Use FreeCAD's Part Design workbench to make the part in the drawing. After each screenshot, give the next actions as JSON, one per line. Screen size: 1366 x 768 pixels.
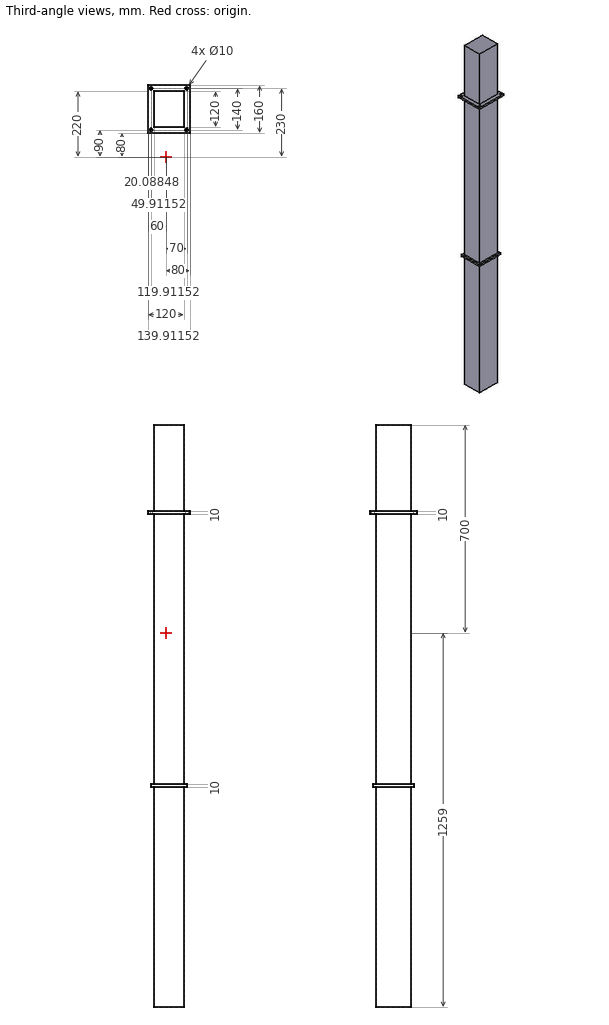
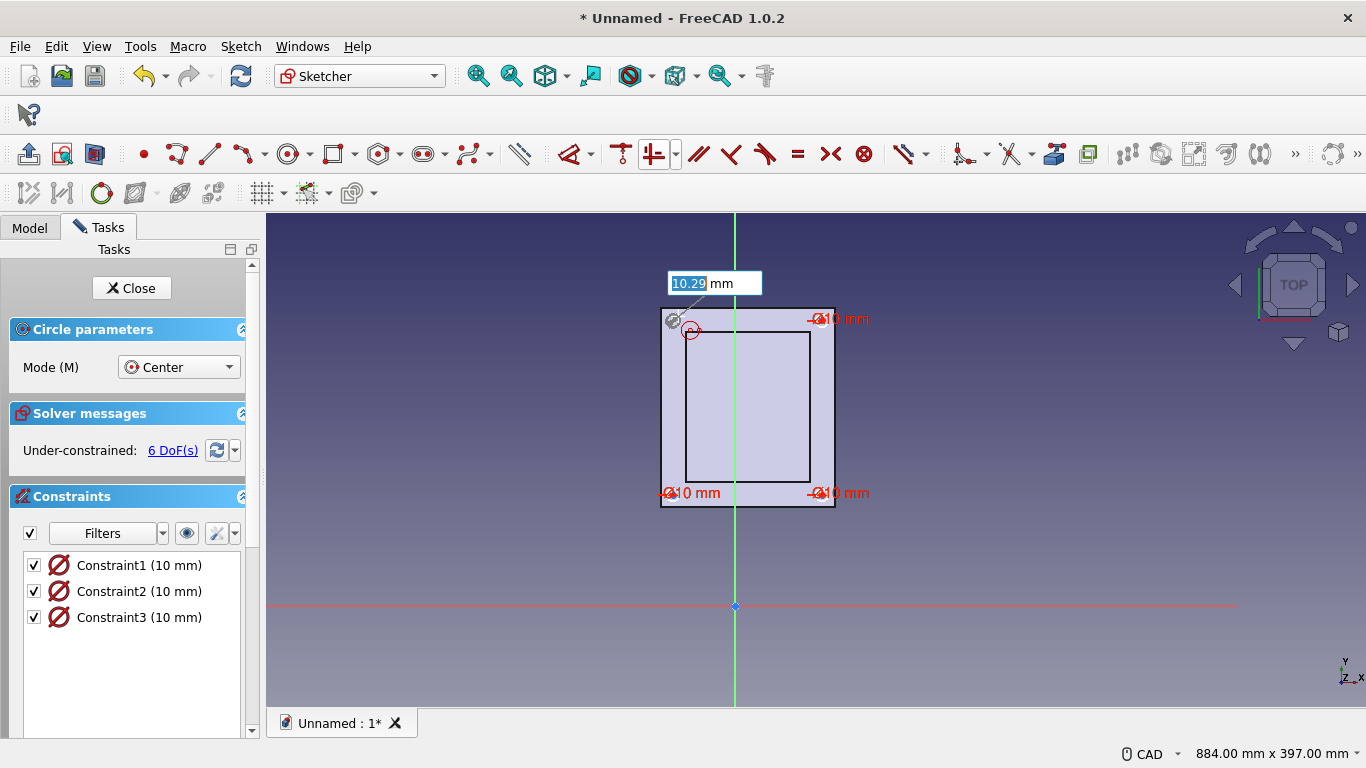
{"action": "type", "text": "10"}
{"action": "key", "text": "Return"}
{"action": "key", "text": "Escape"}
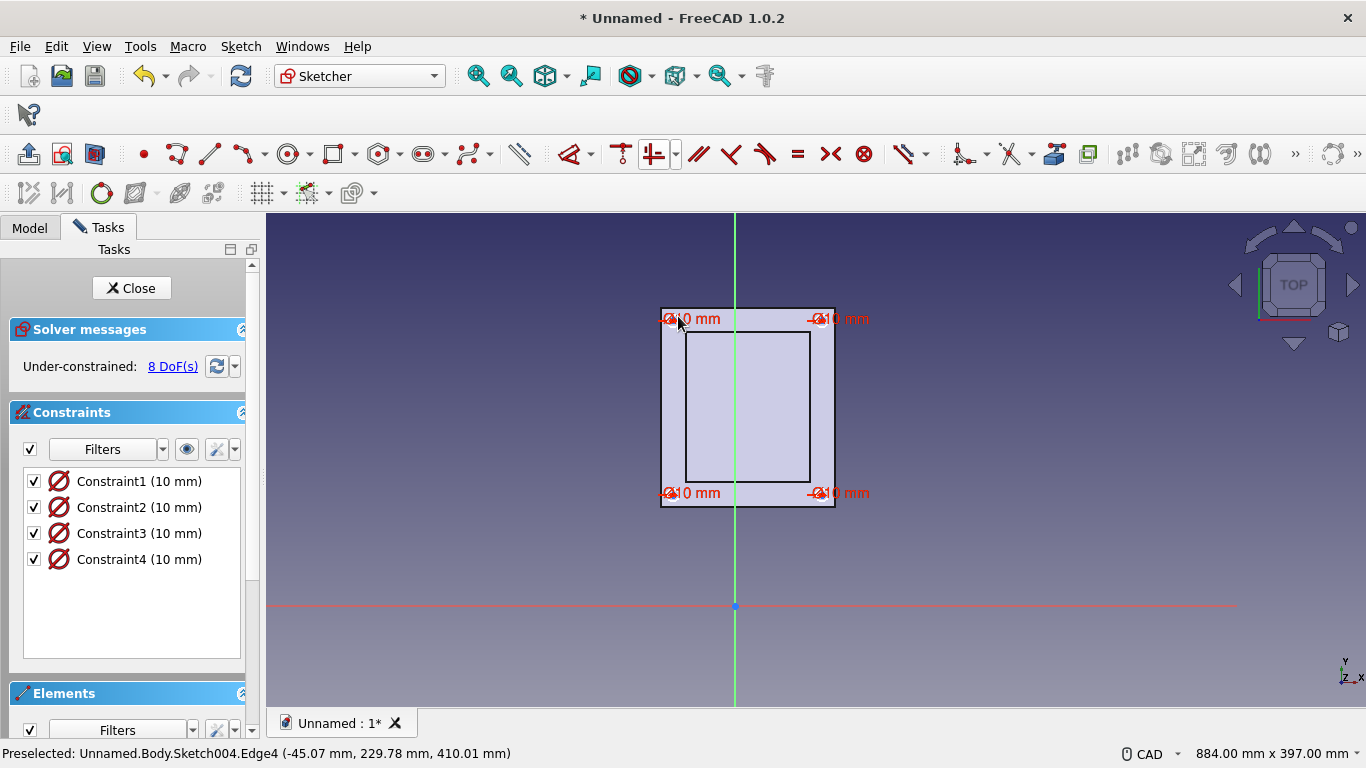
{"action": "left_click", "coordinate": [822, 321]}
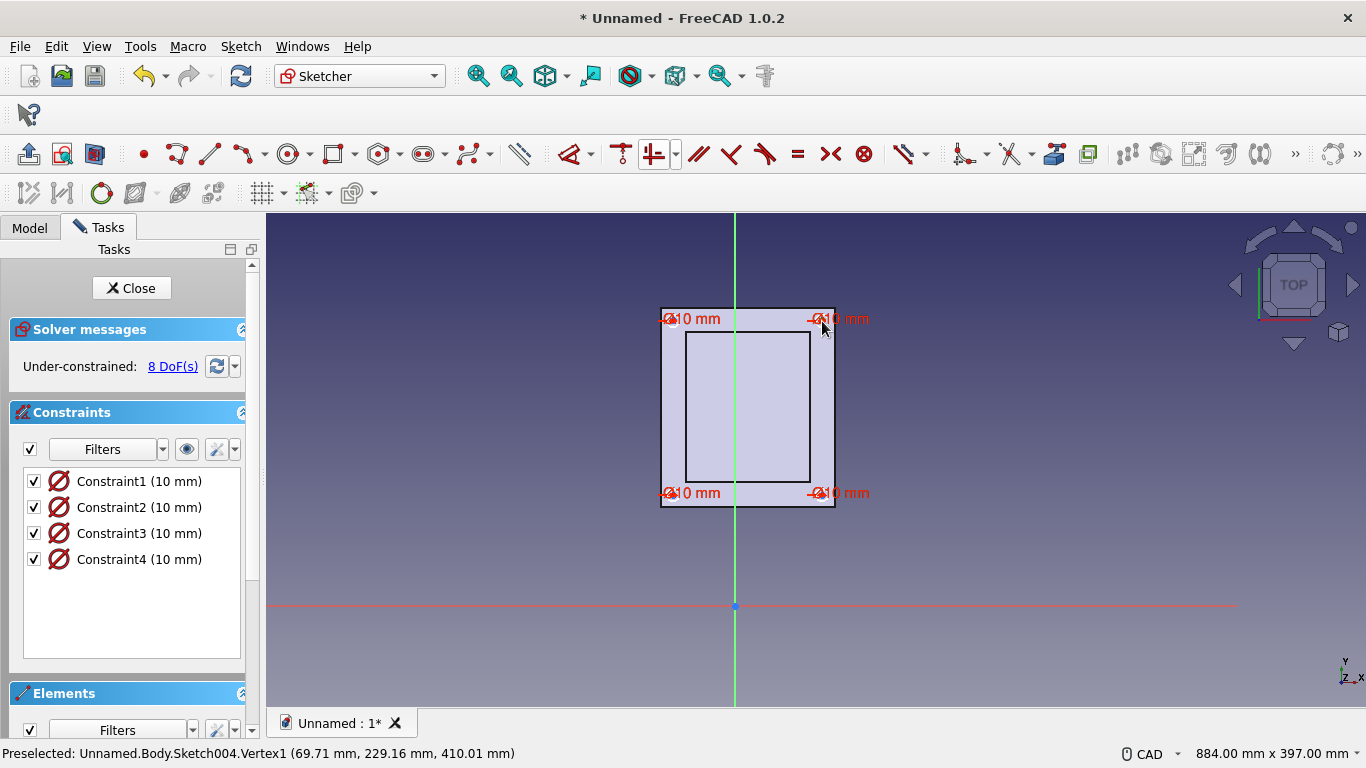
{"action": "left_click", "coordinate": [822, 495]}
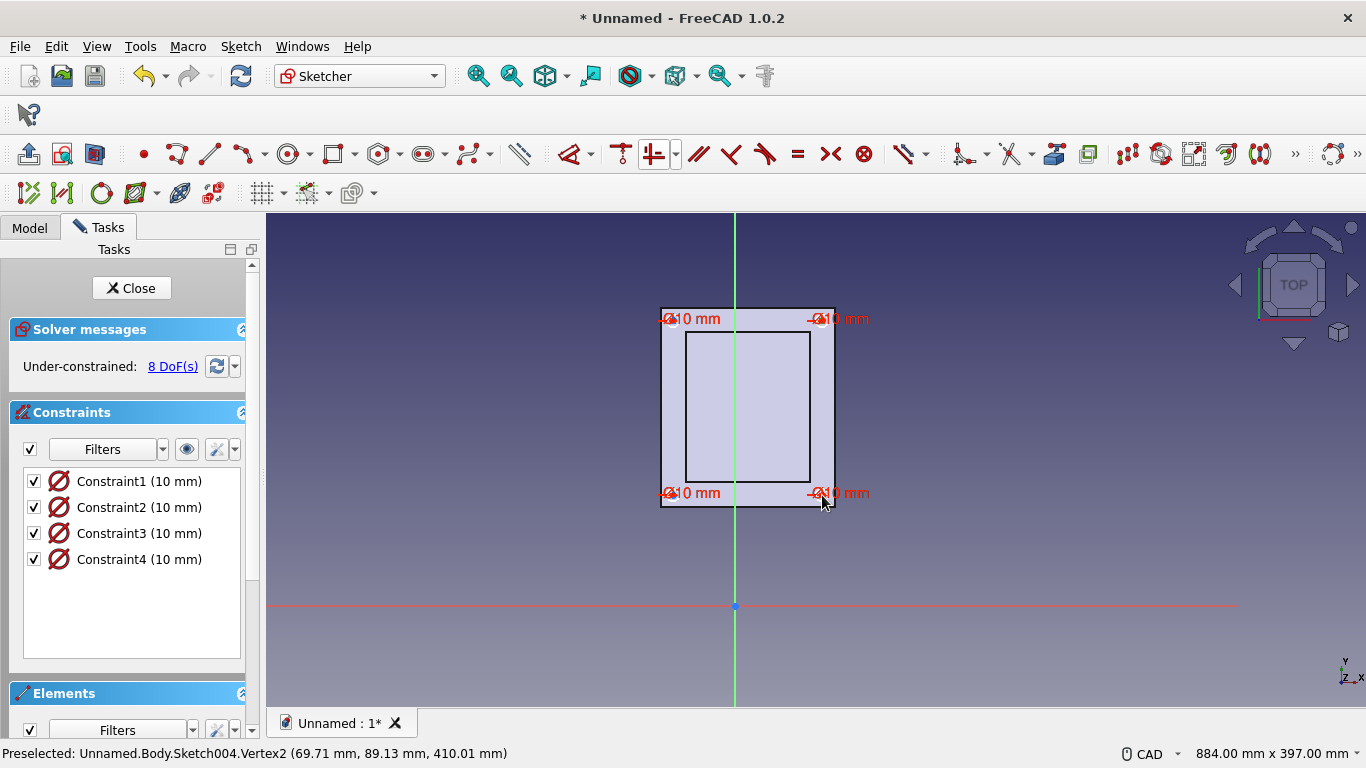
{"action": "key", "text": "v"}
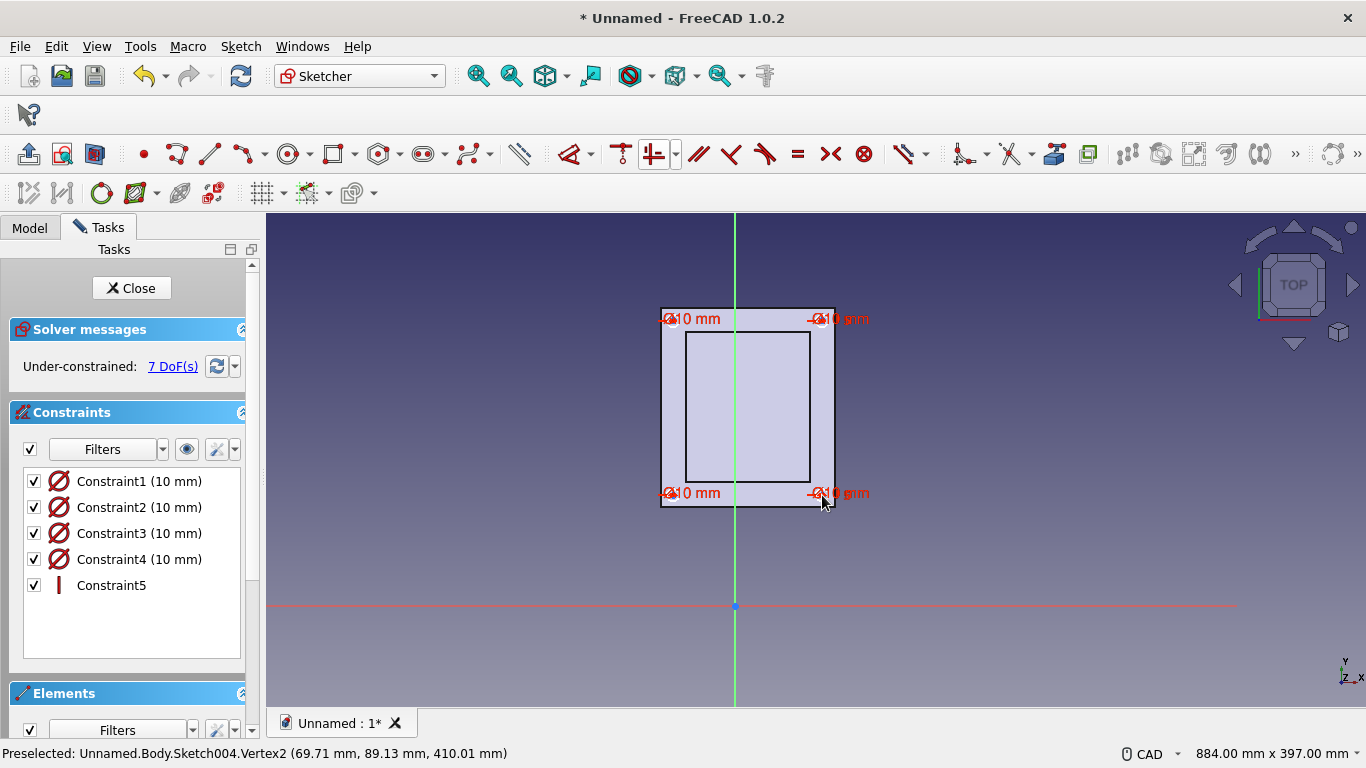
{"action": "left_click", "coordinate": [822, 495]}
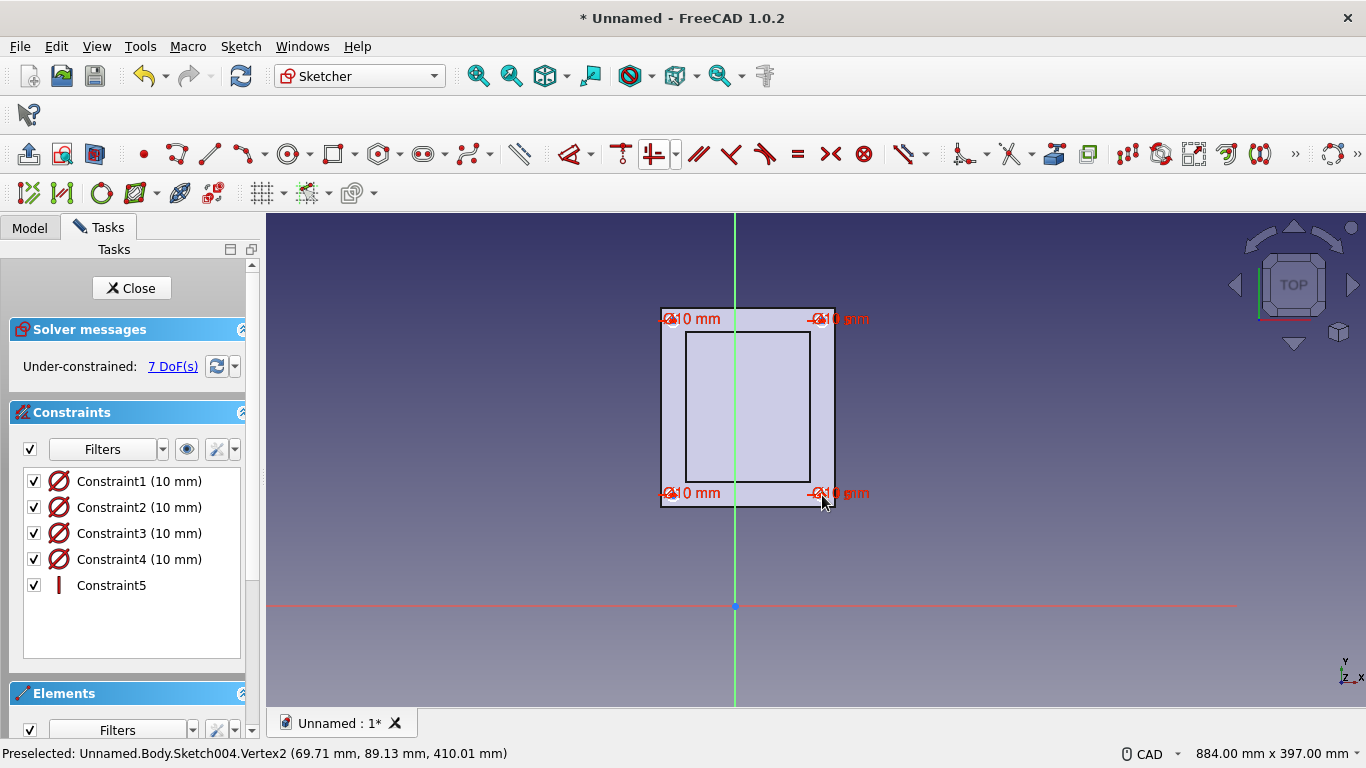
{"action": "left_click", "coordinate": [673, 495]}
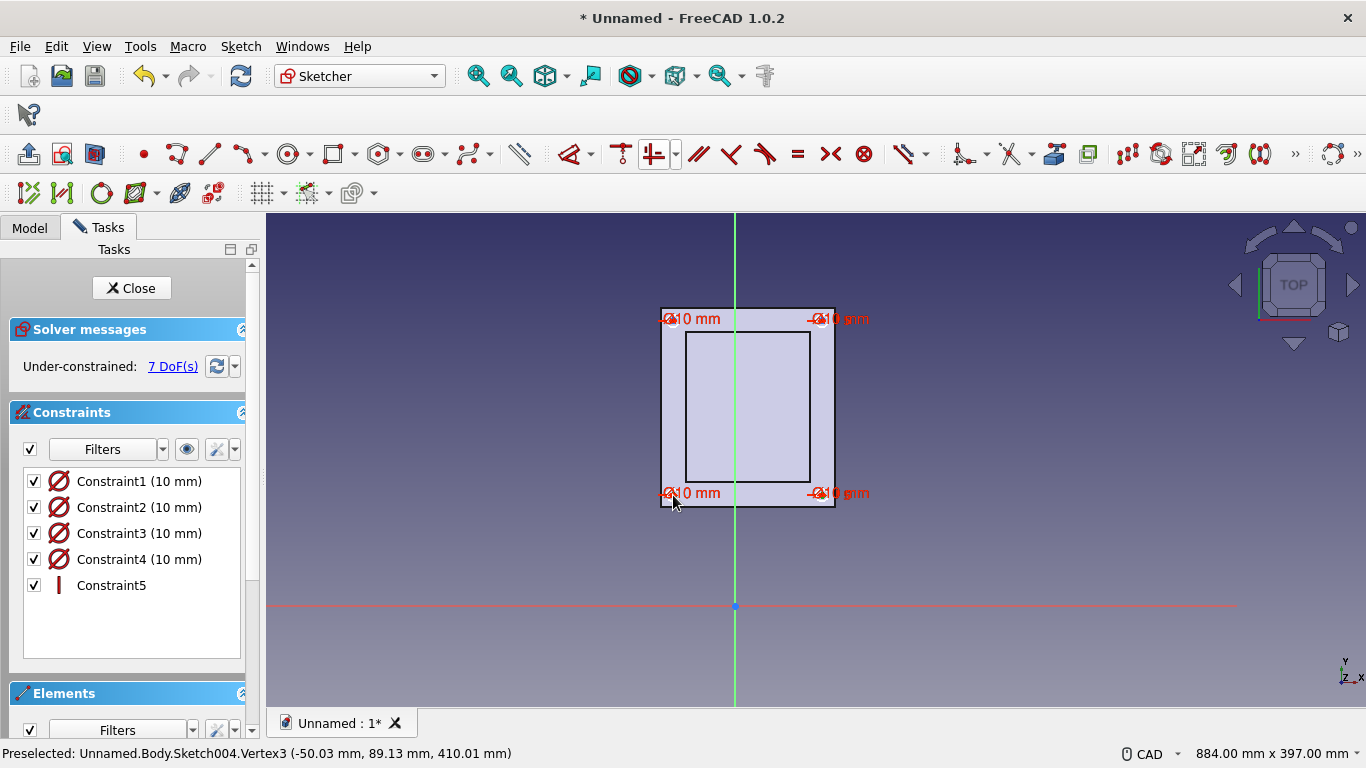
{"action": "key", "text": "h"}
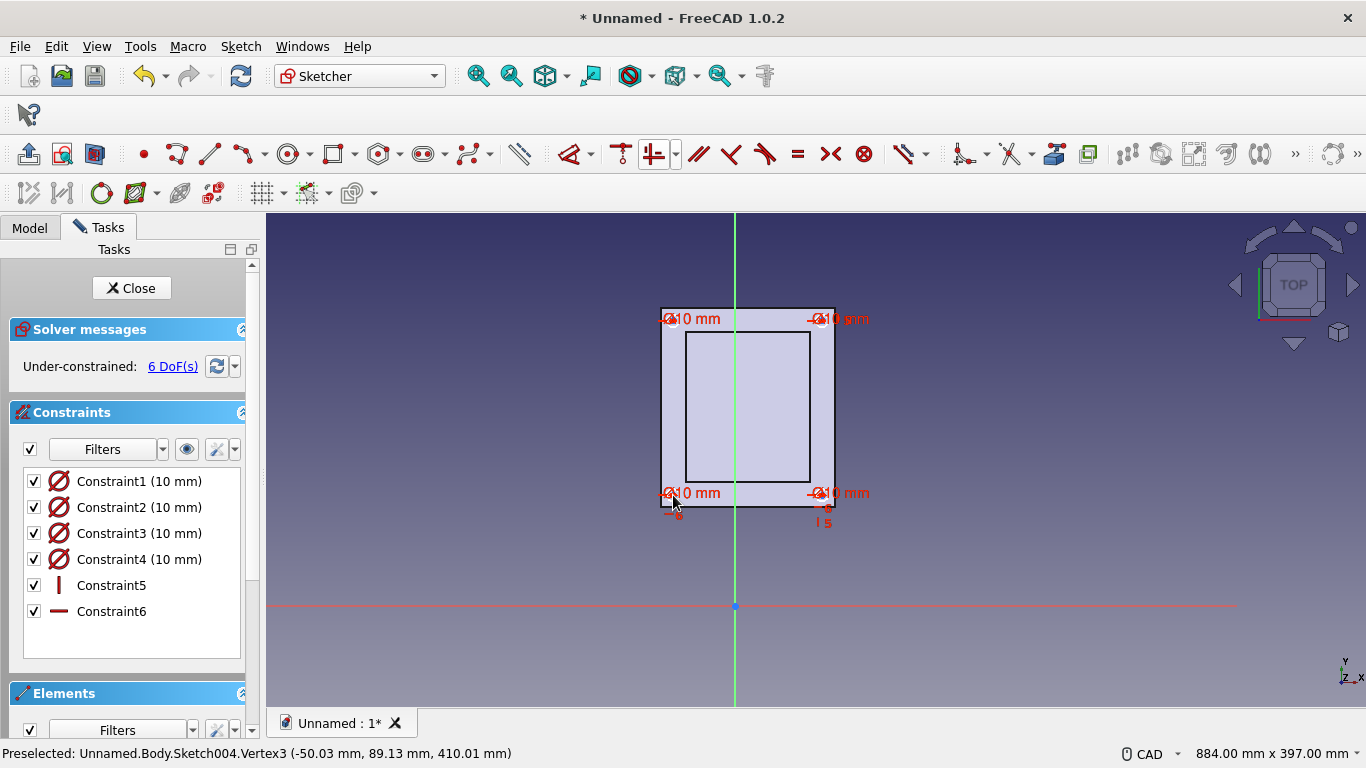
{"action": "left_click", "coordinate": [673, 495]}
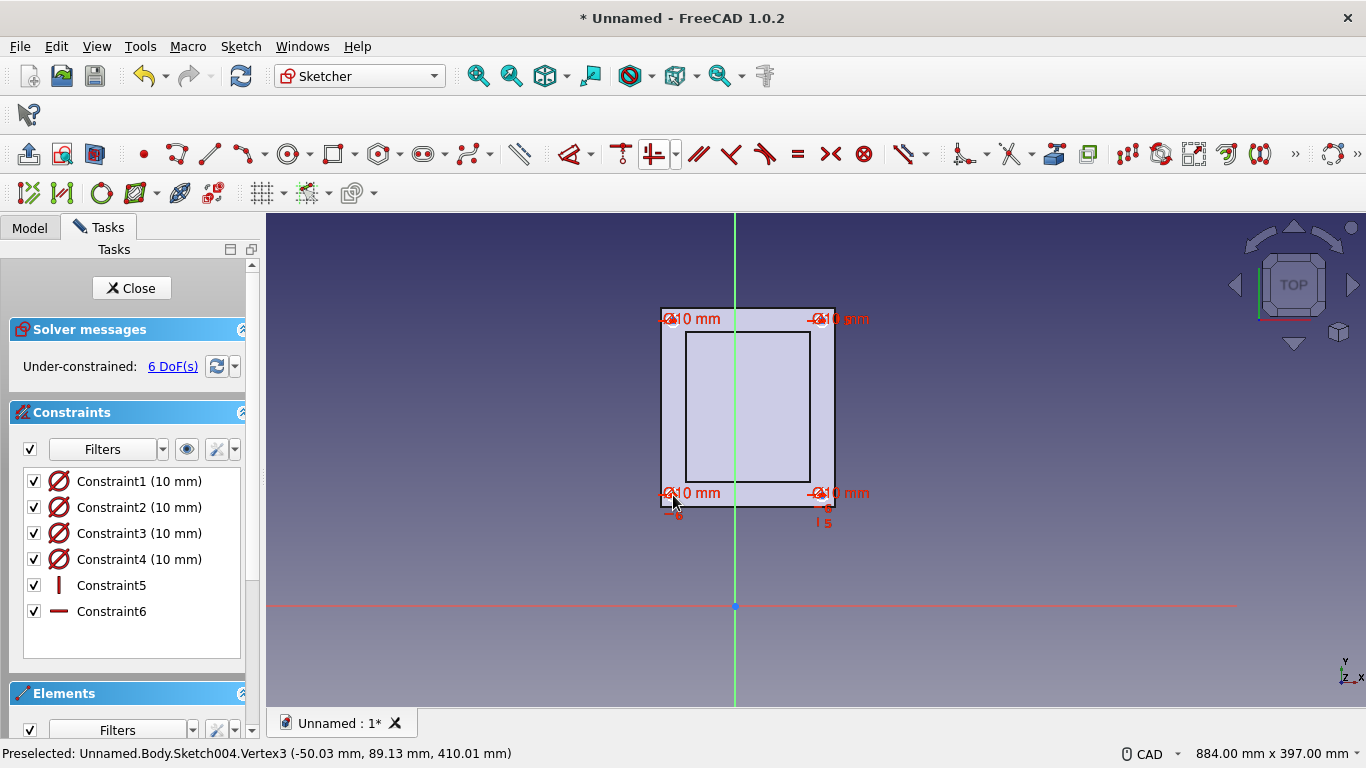
{"action": "left_click", "coordinate": [673, 321]}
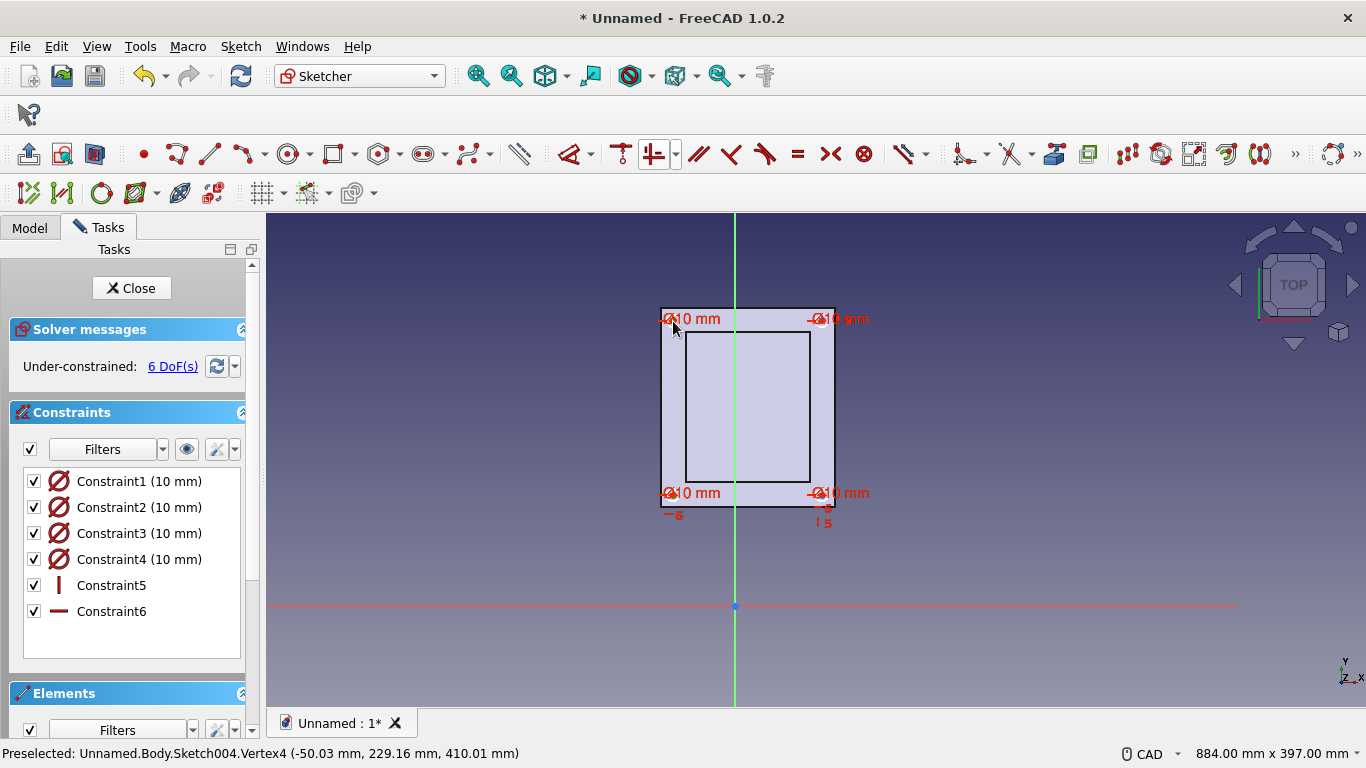
{"action": "left_click", "coordinate": [676, 154]}